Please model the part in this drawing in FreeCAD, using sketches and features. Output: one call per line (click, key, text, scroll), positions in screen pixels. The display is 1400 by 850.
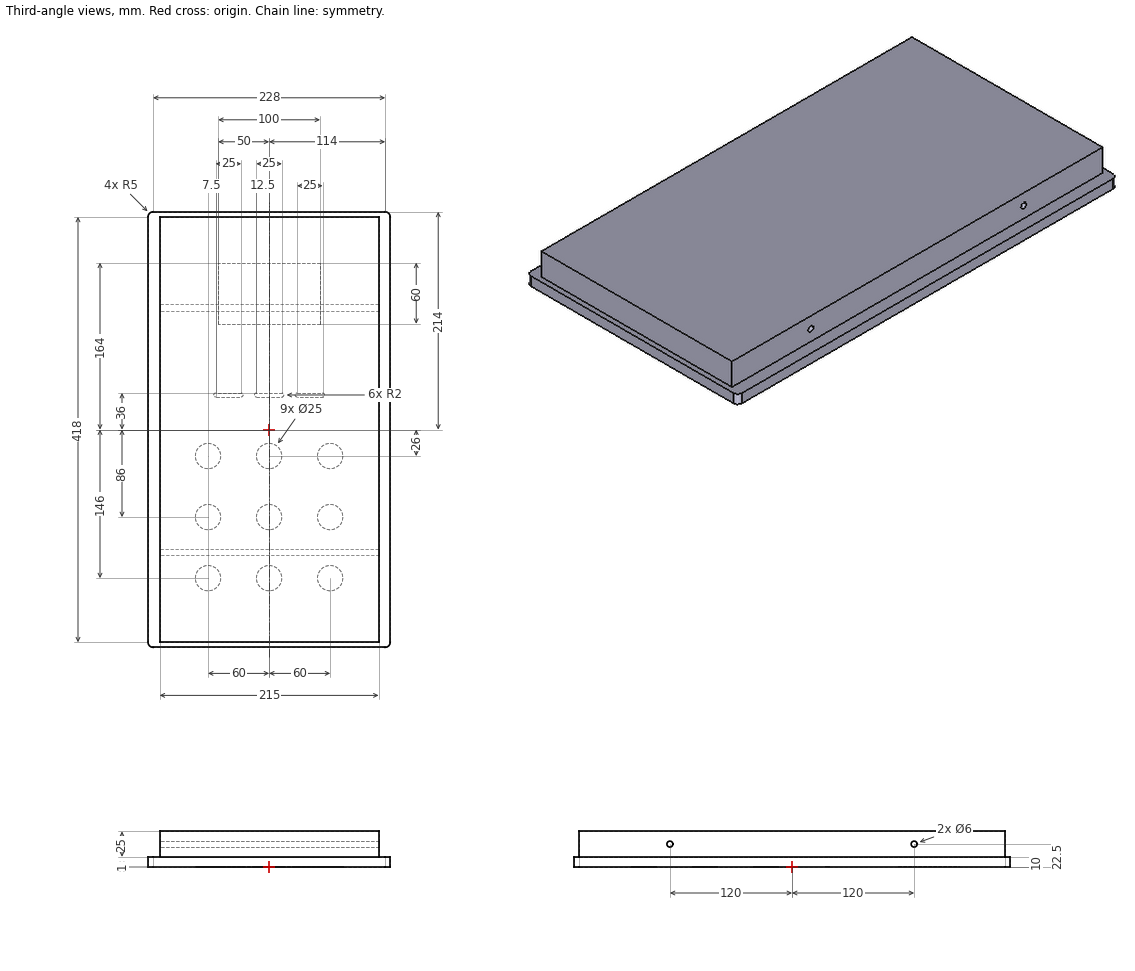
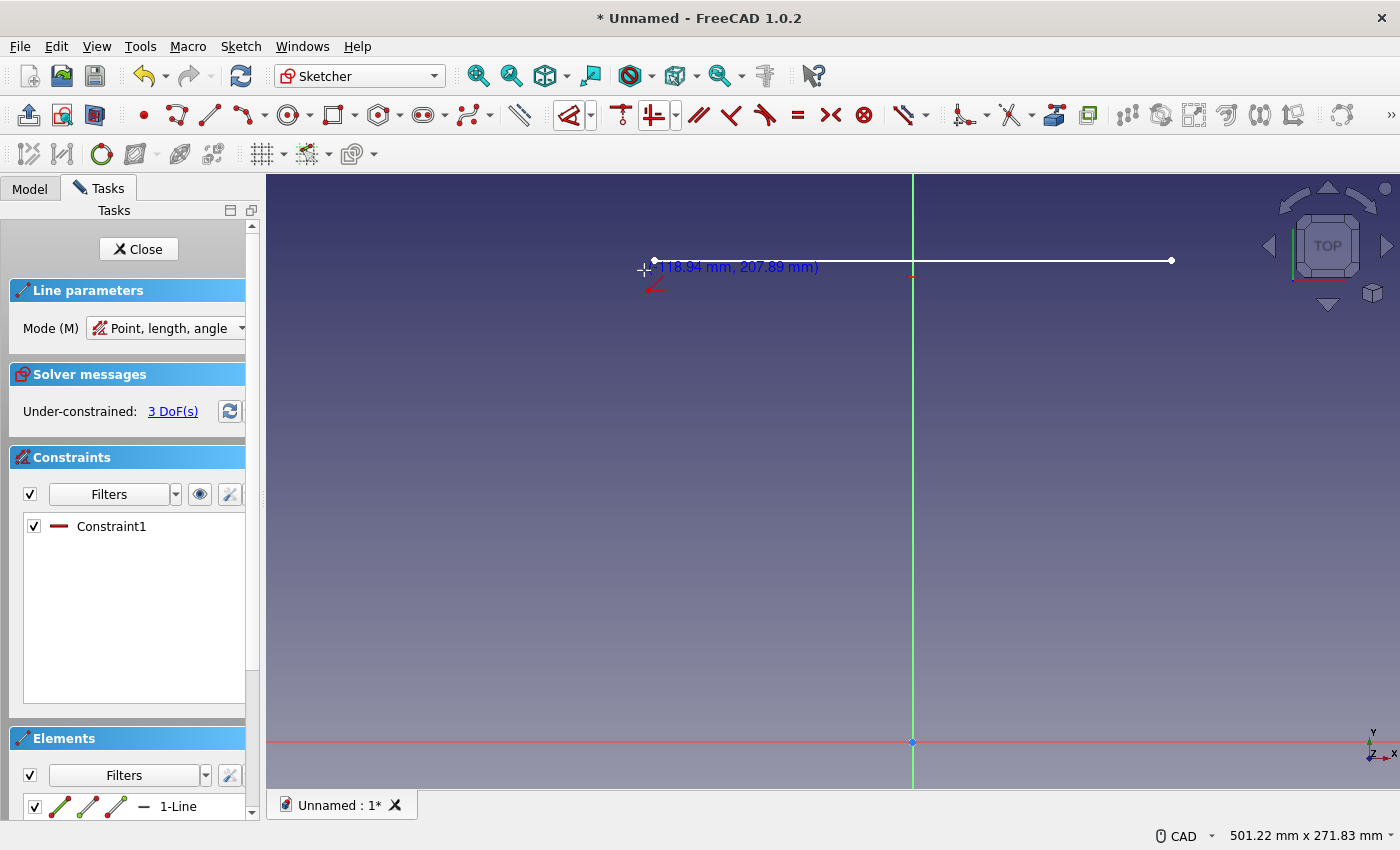
click(643, 270)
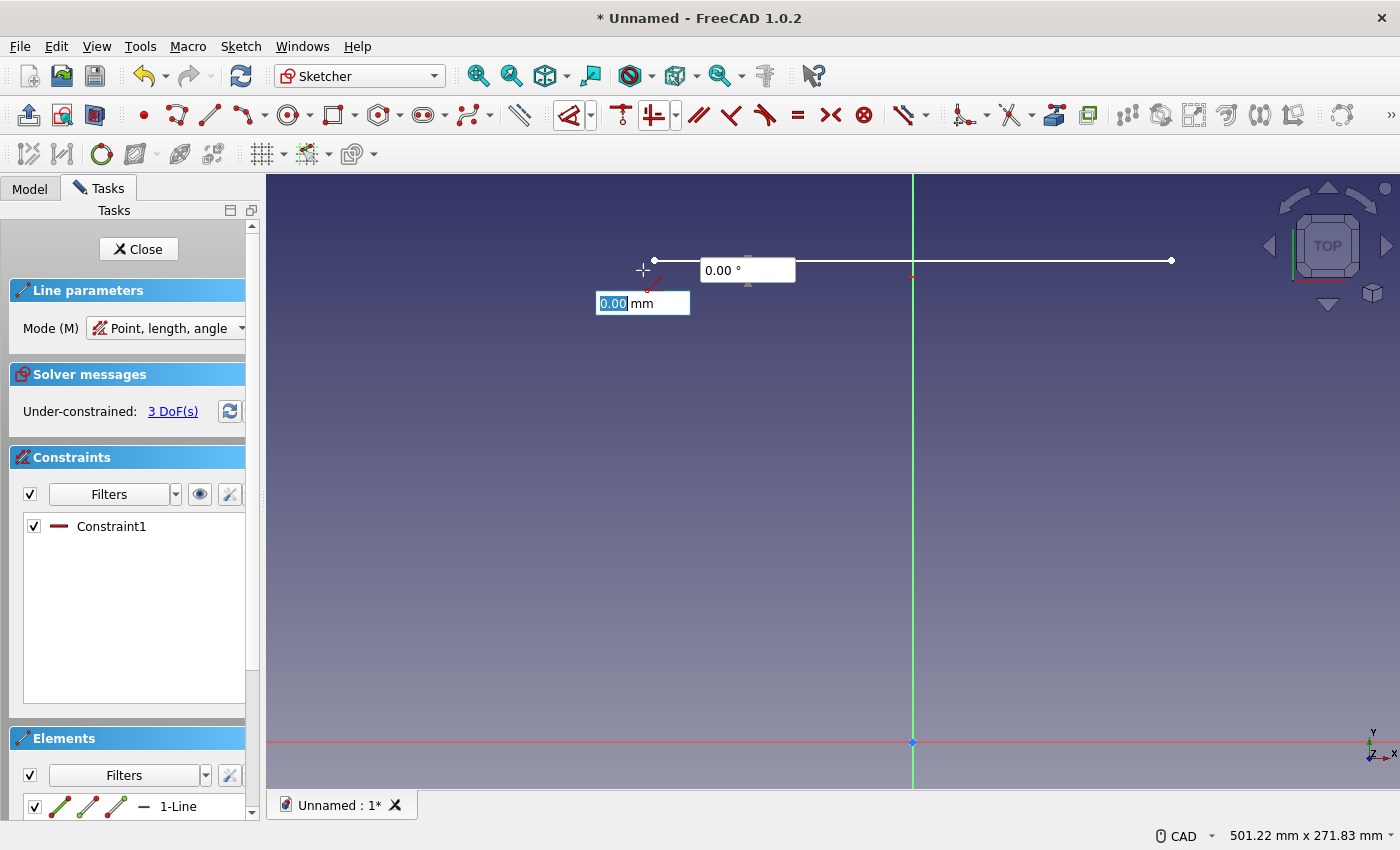
scroll(644, 269, down, 4)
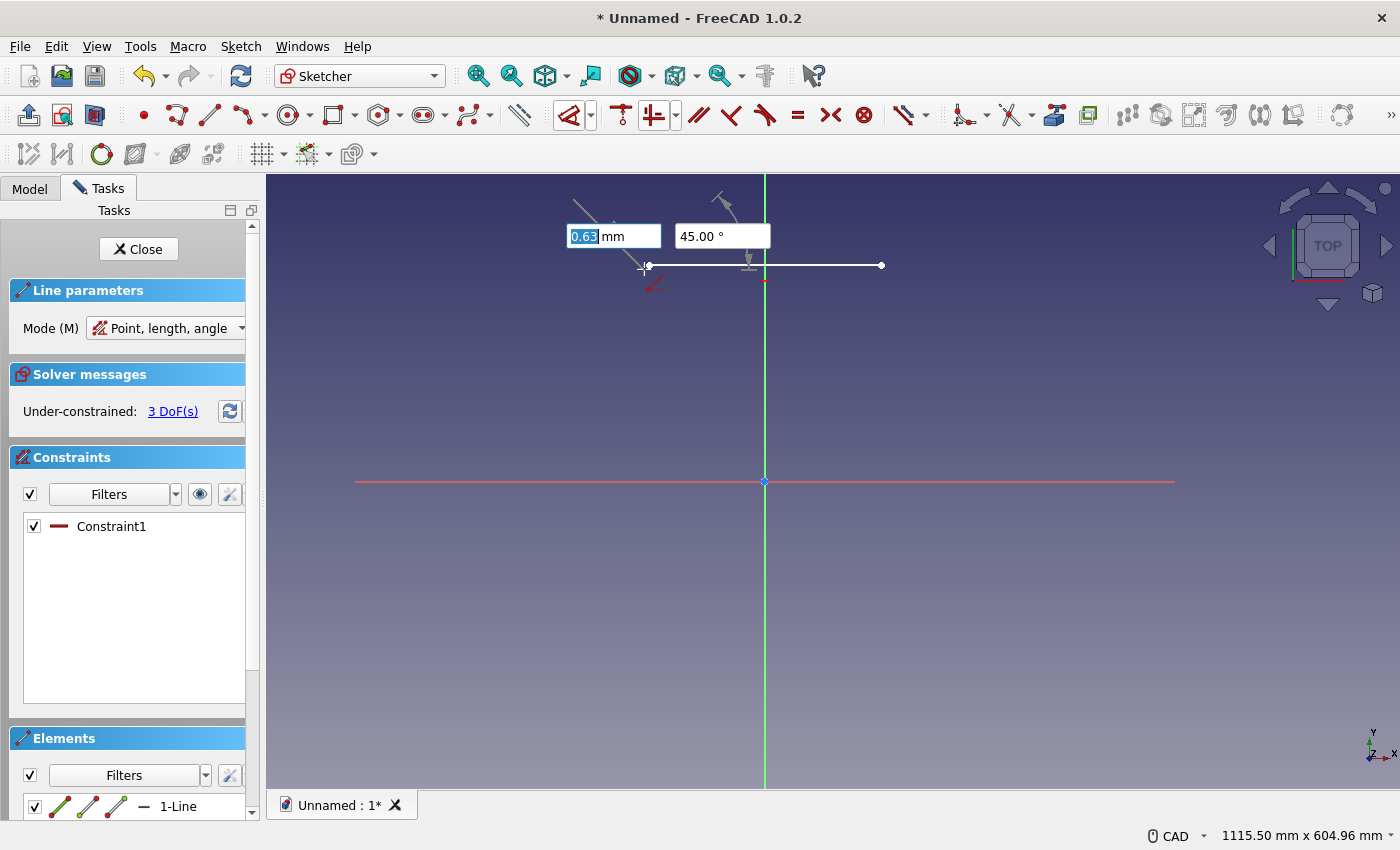
click(644, 694)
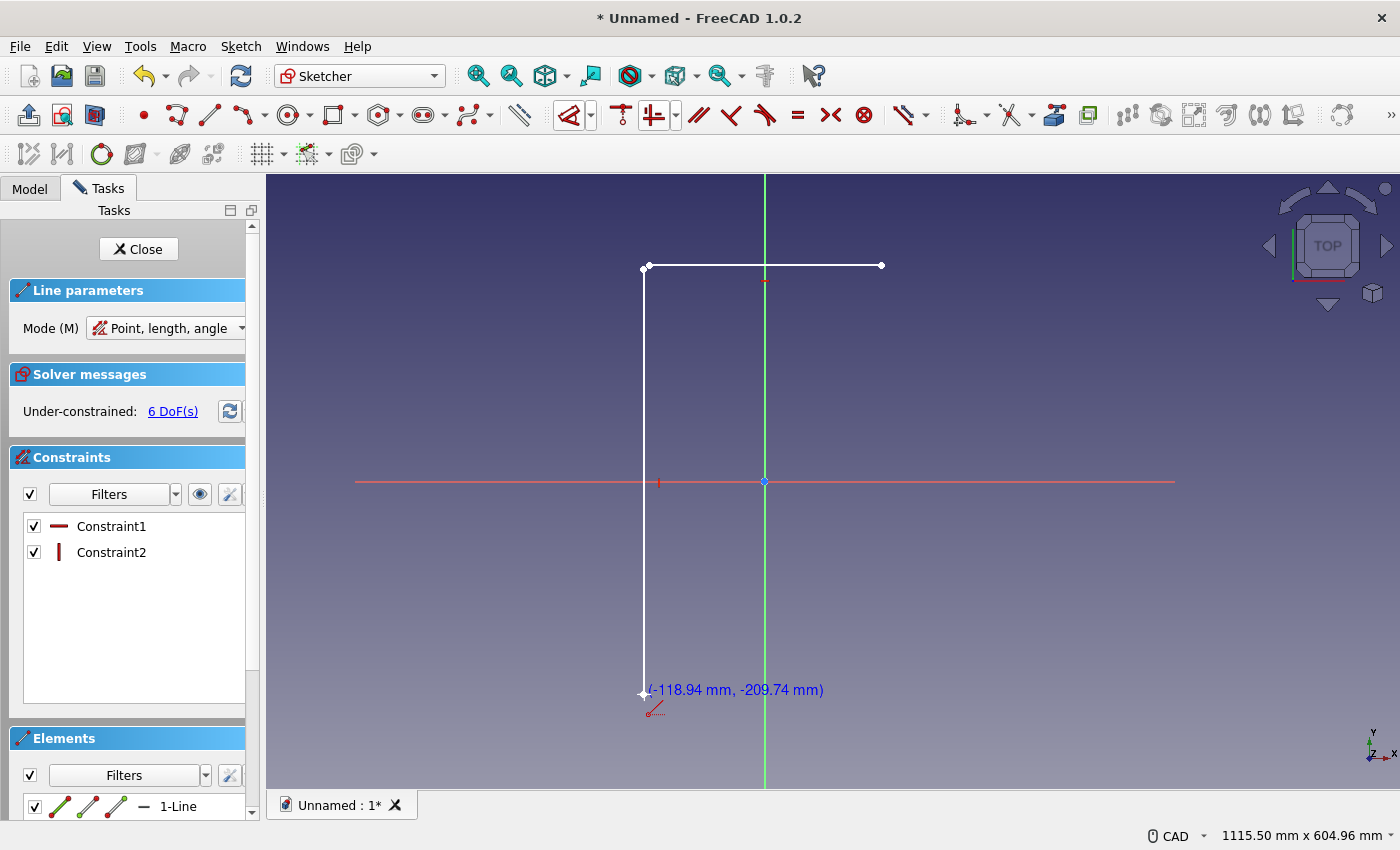
scroll(649, 699, up, 4)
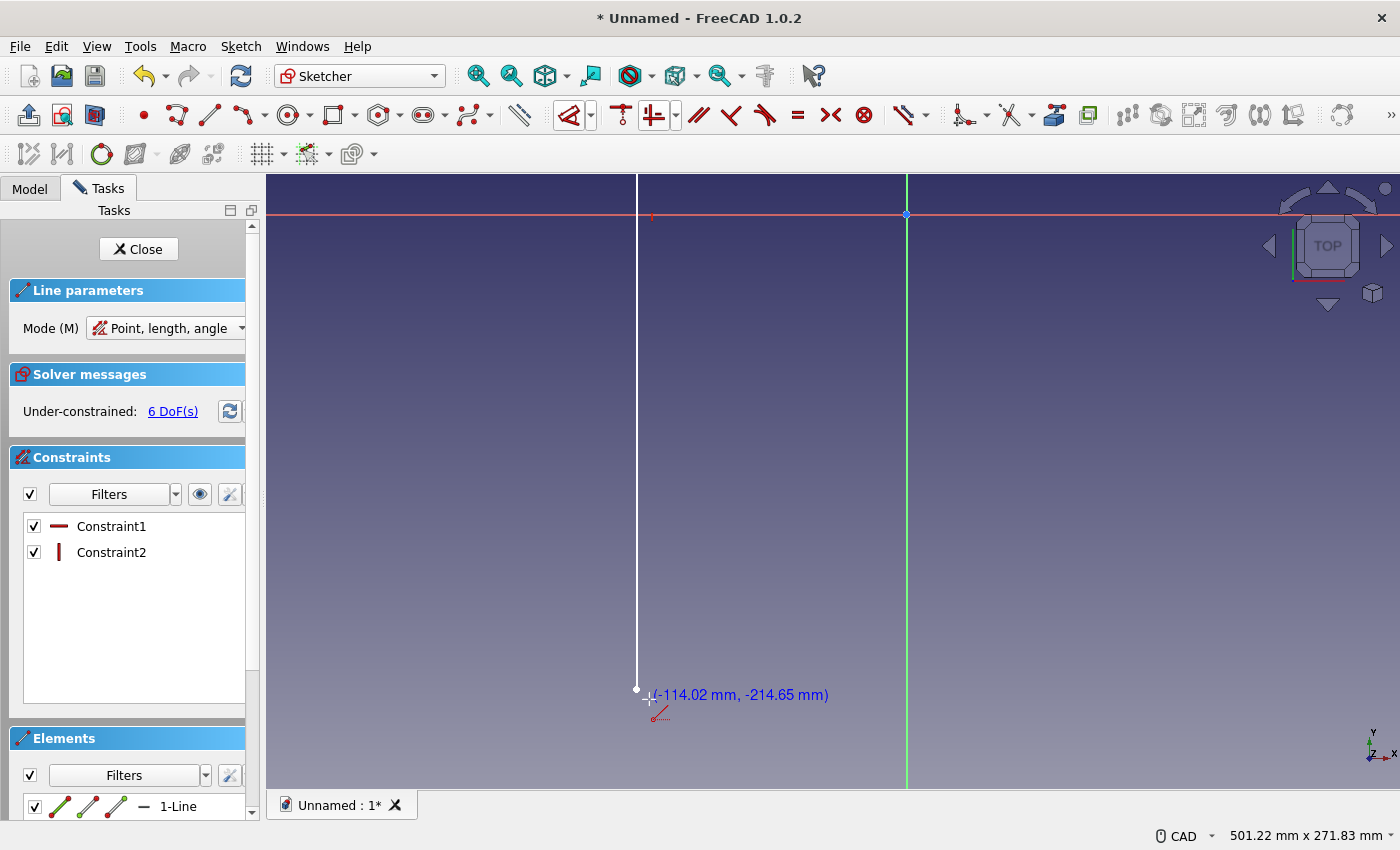
click(649, 699)
click(1164, 699)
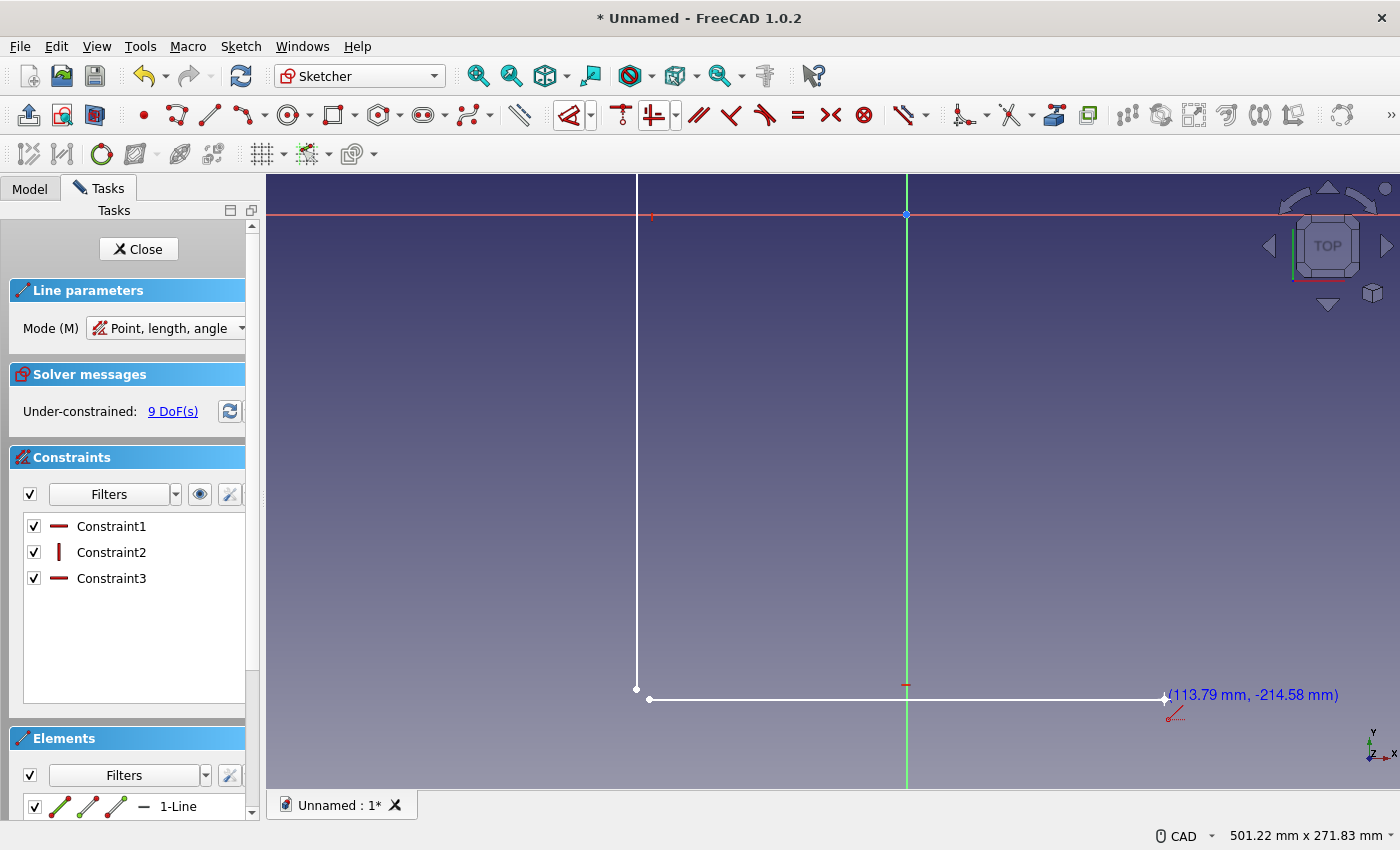
click(1176, 687)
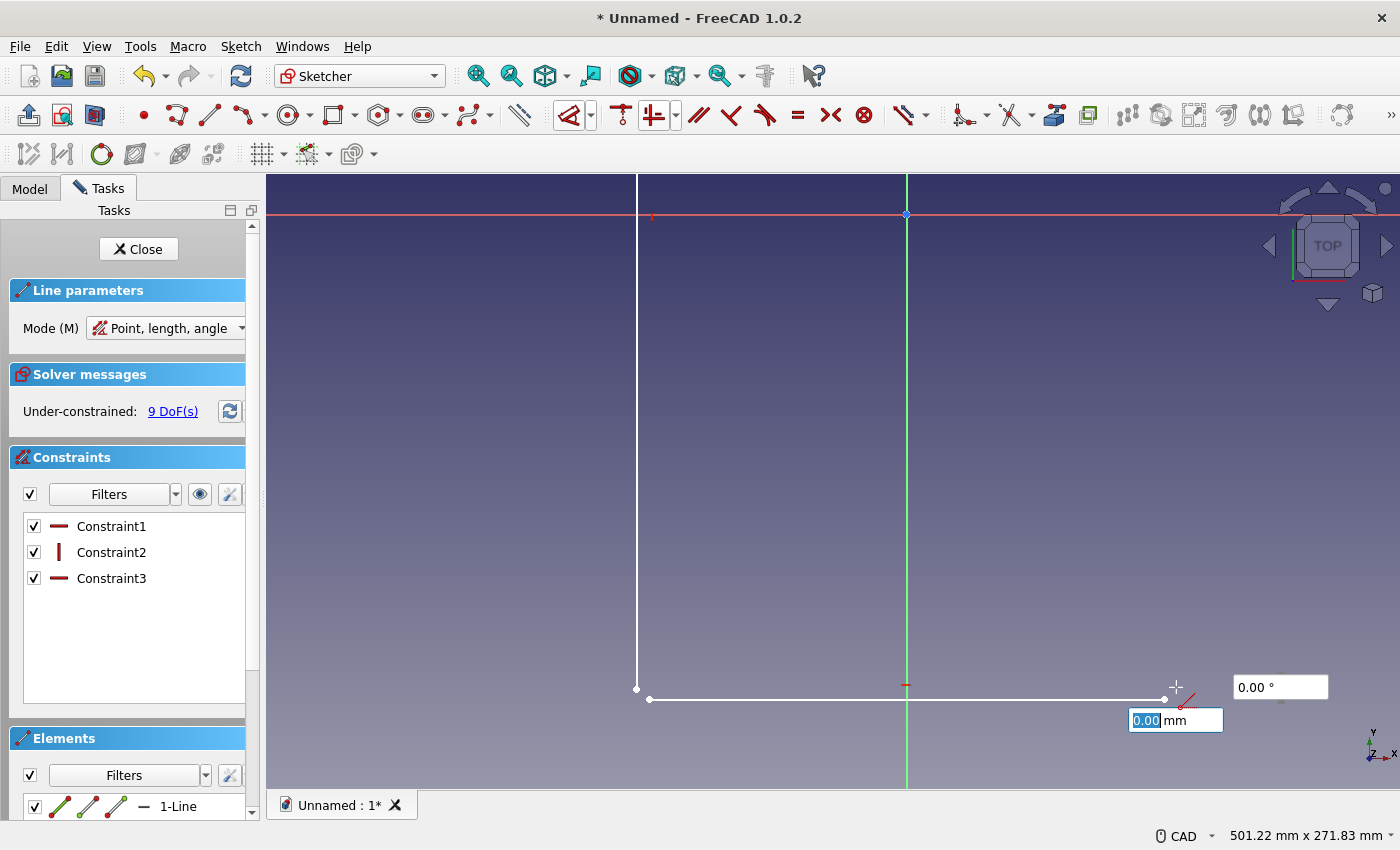
scroll(649, 699, down, 4)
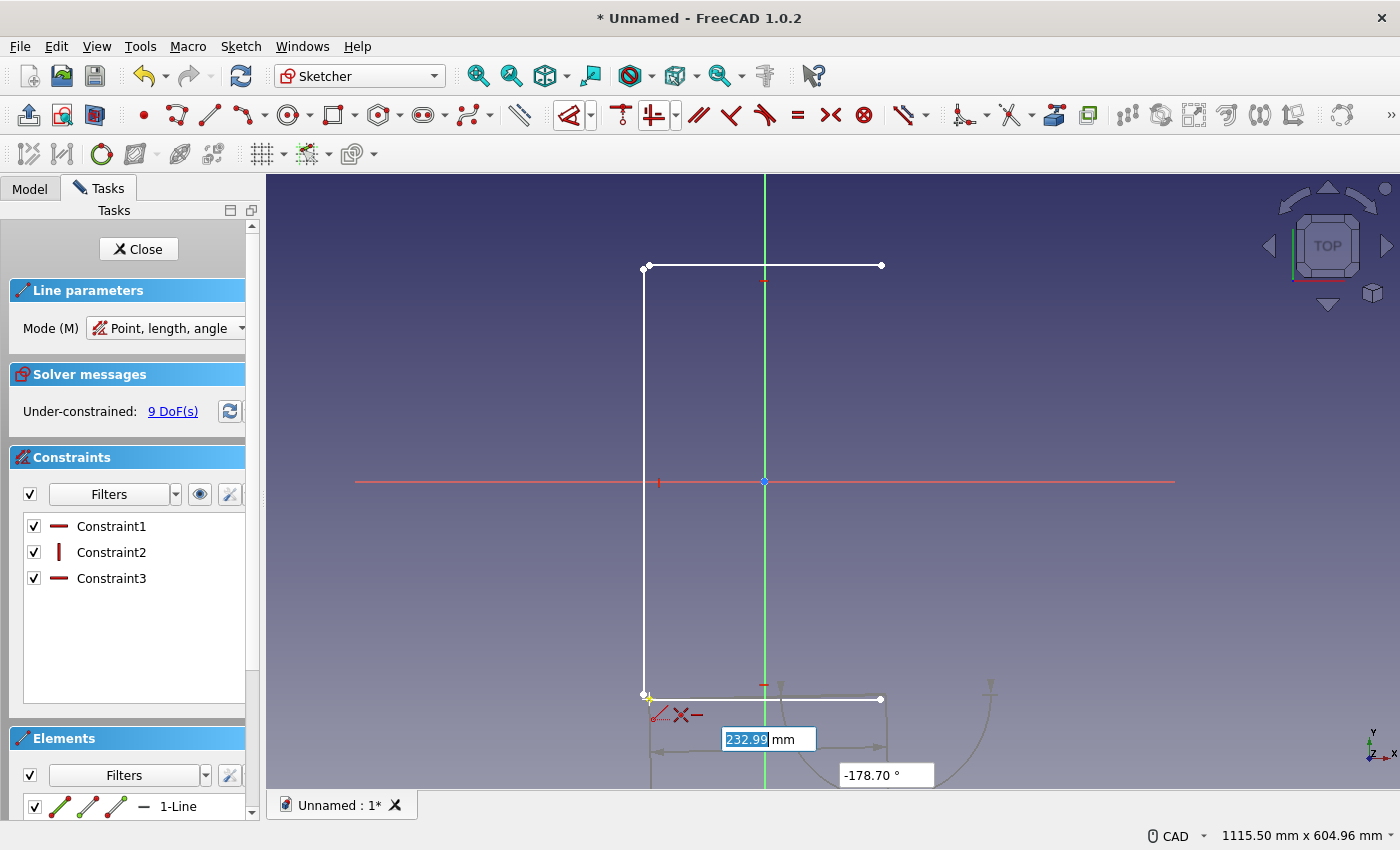
scroll(886, 269, up, 4)